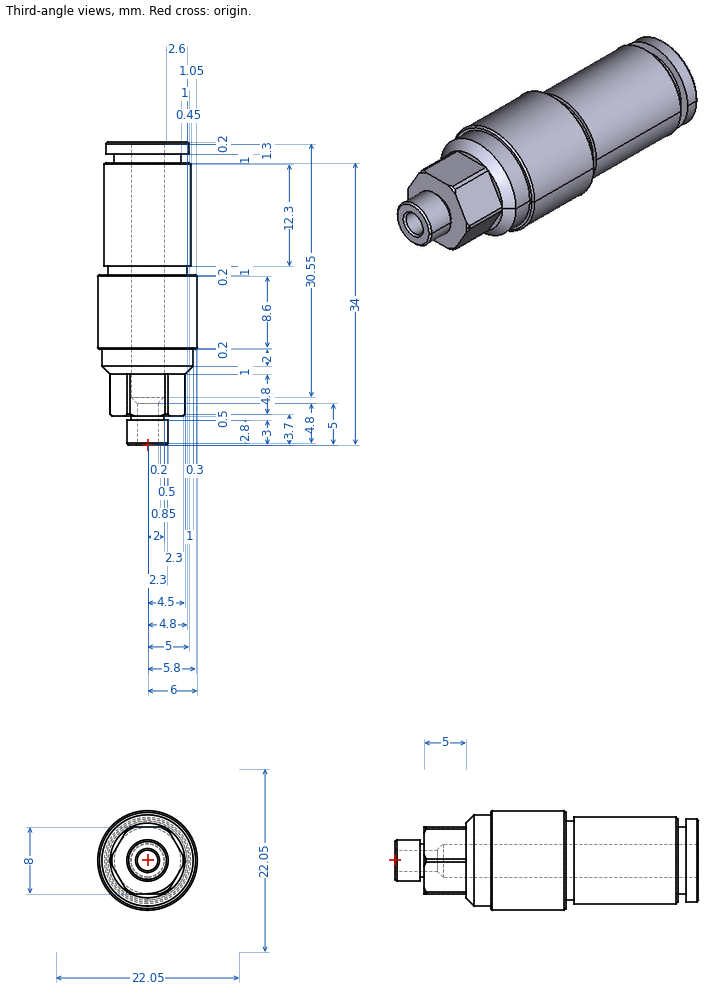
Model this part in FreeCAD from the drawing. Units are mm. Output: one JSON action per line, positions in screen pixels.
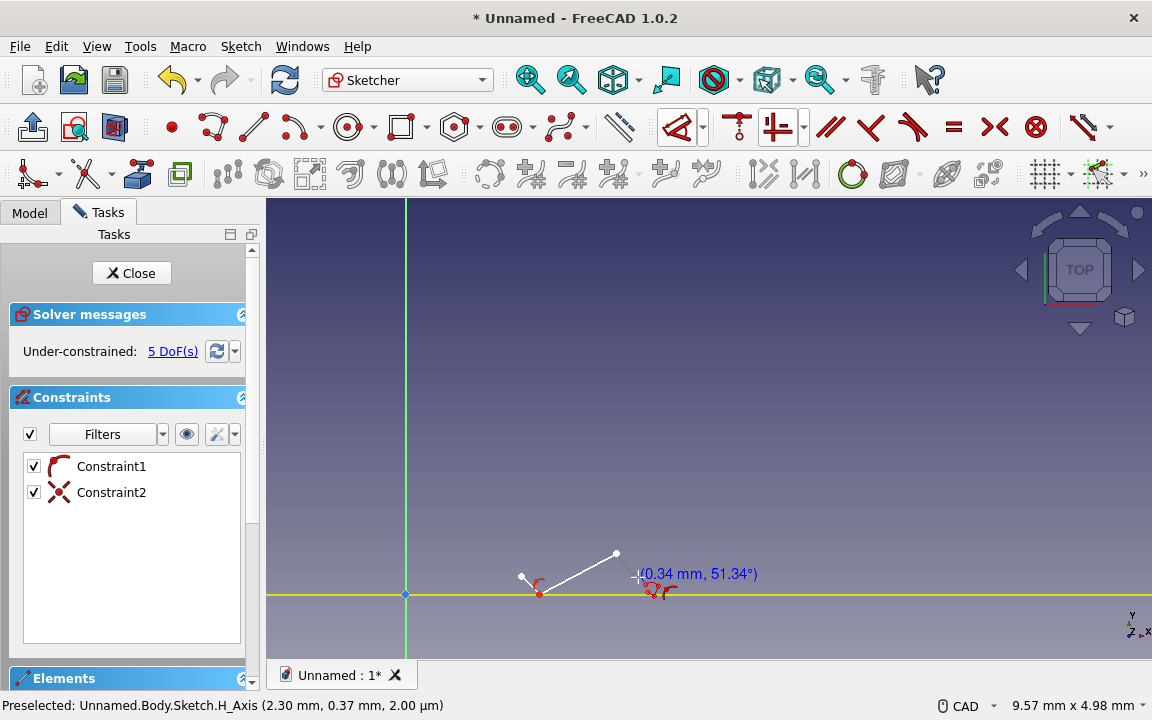
{"action": "left_click", "coordinate": [637, 576]}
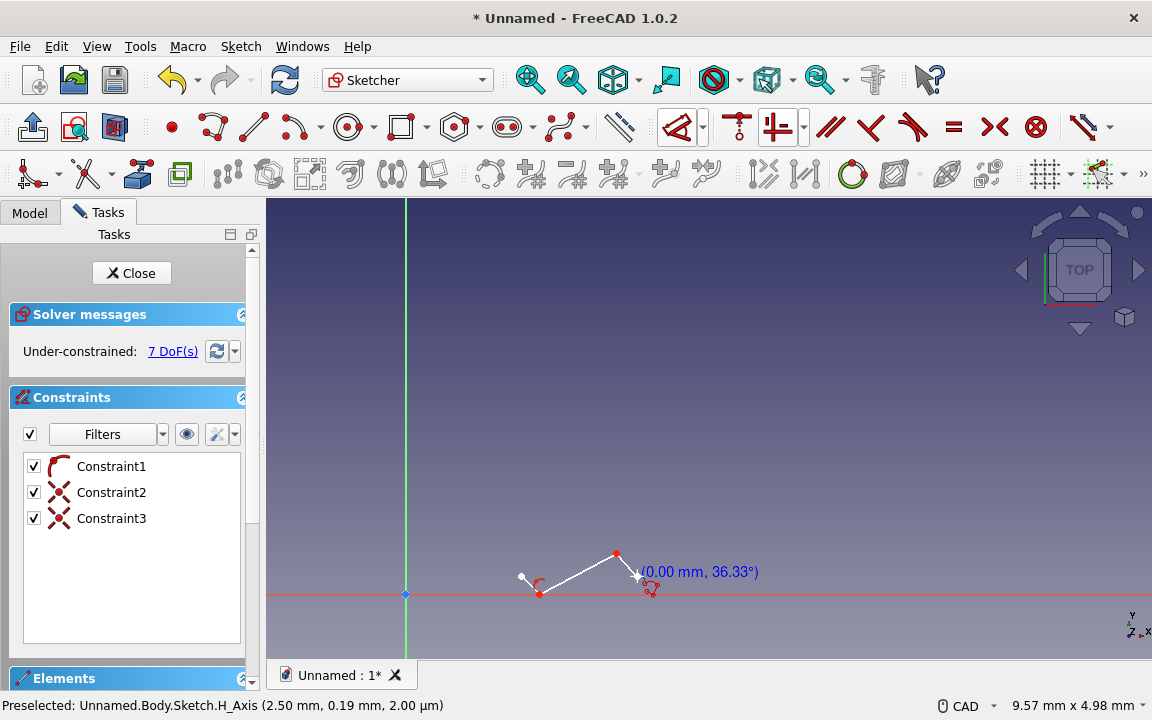
{"action": "scroll", "coordinate": [636, 581], "scroll_direction": "down", "scroll_amount": 12}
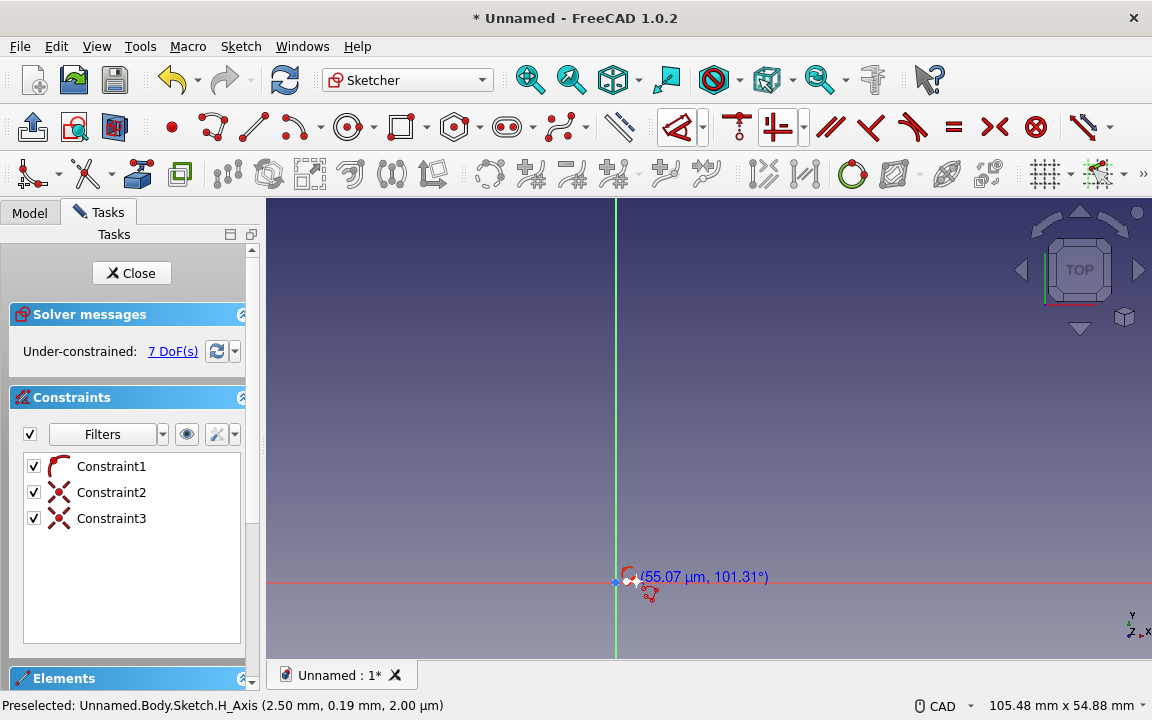
{"action": "left_click", "coordinate": [636, 558]}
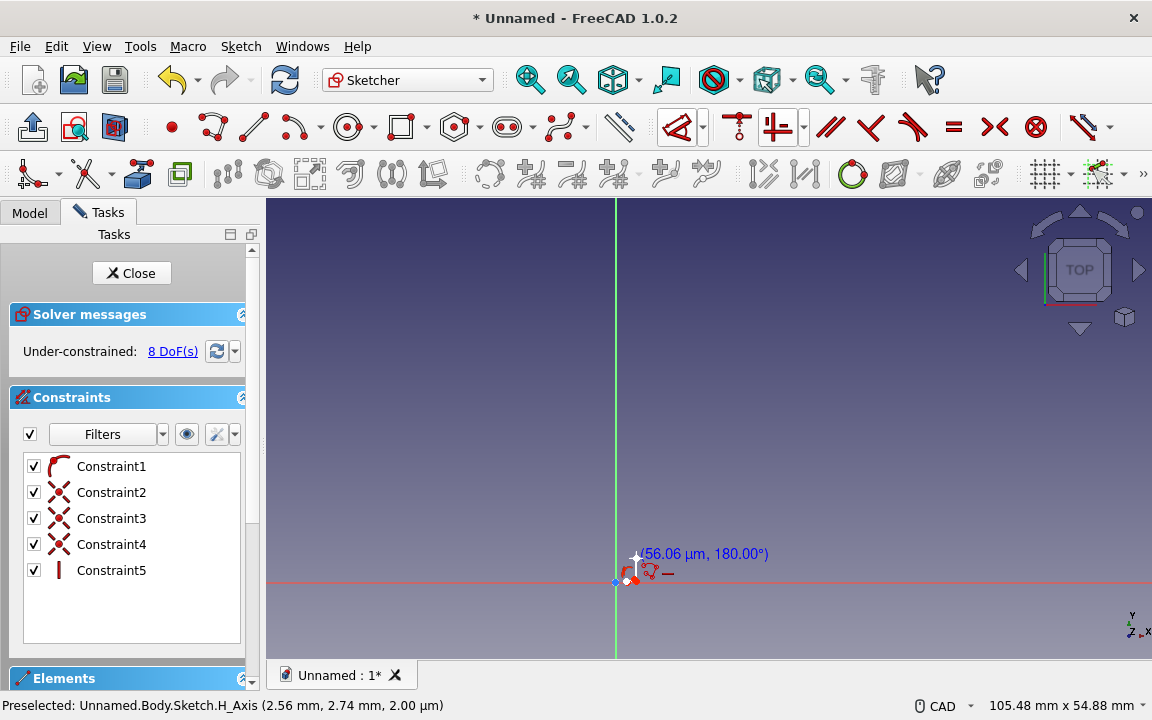
{"action": "scroll", "coordinate": [632, 558], "scroll_direction": "up", "scroll_amount": 7}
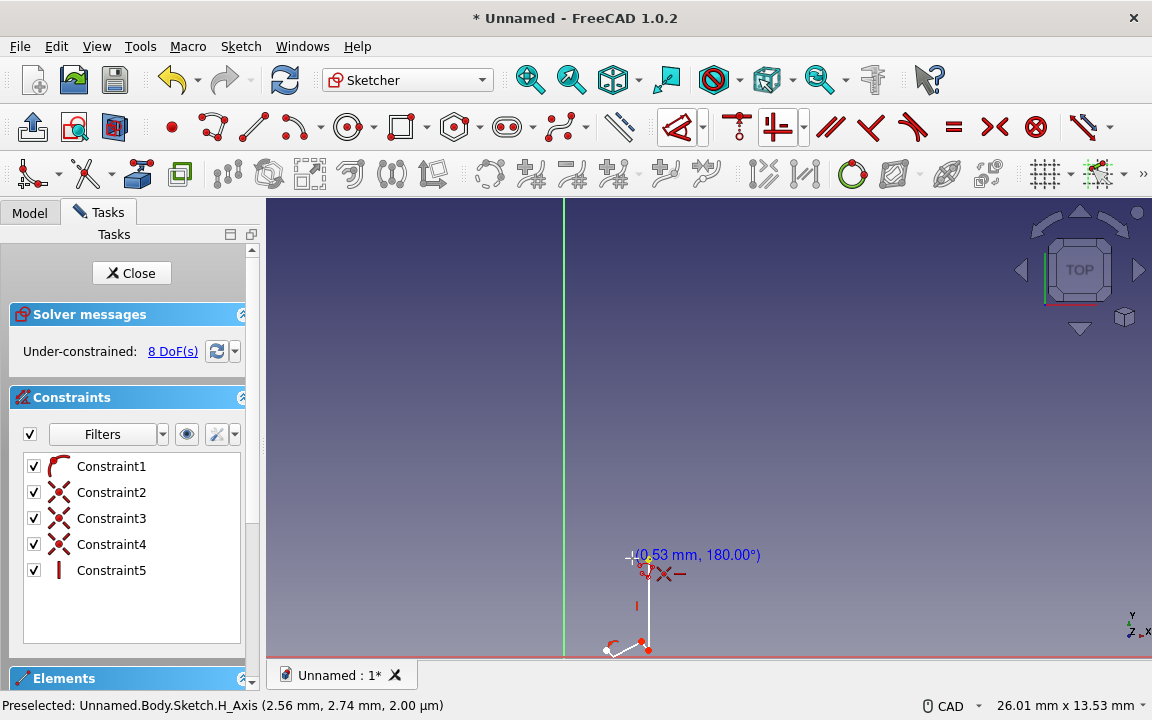
{"action": "left_click", "coordinate": [632, 556]}
{"action": "left_click", "coordinate": [632, 538]}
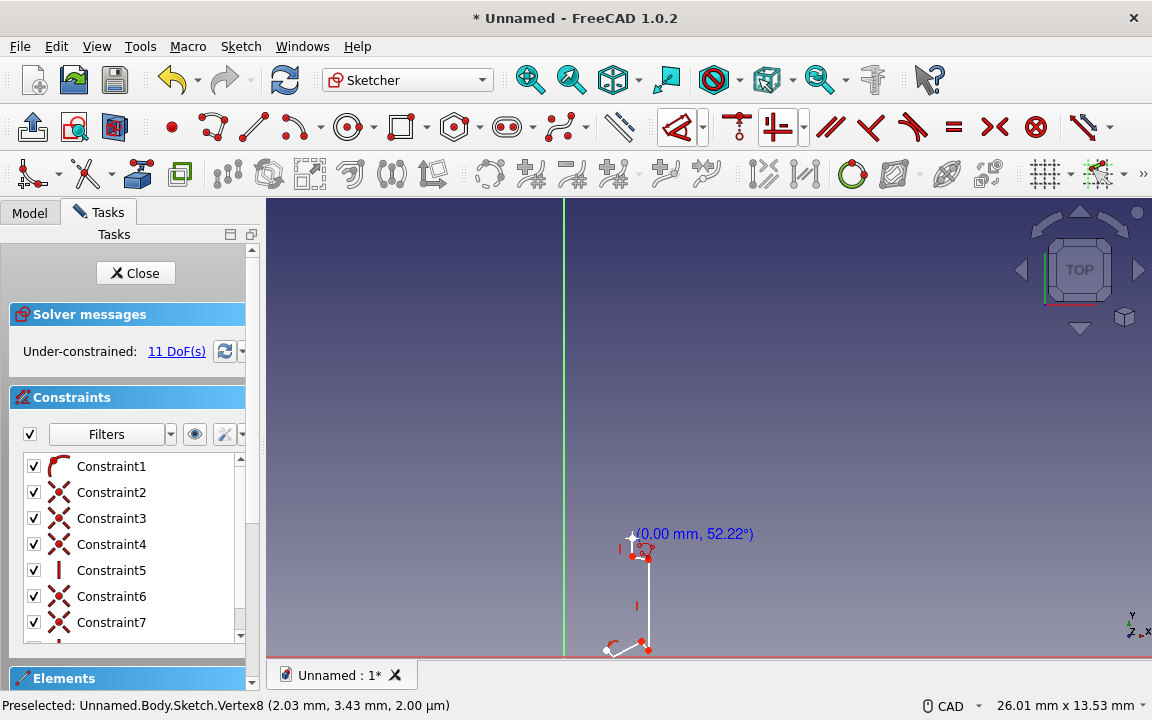
{"action": "scroll", "coordinate": [632, 557], "scroll_direction": "down", "scroll_amount": 7}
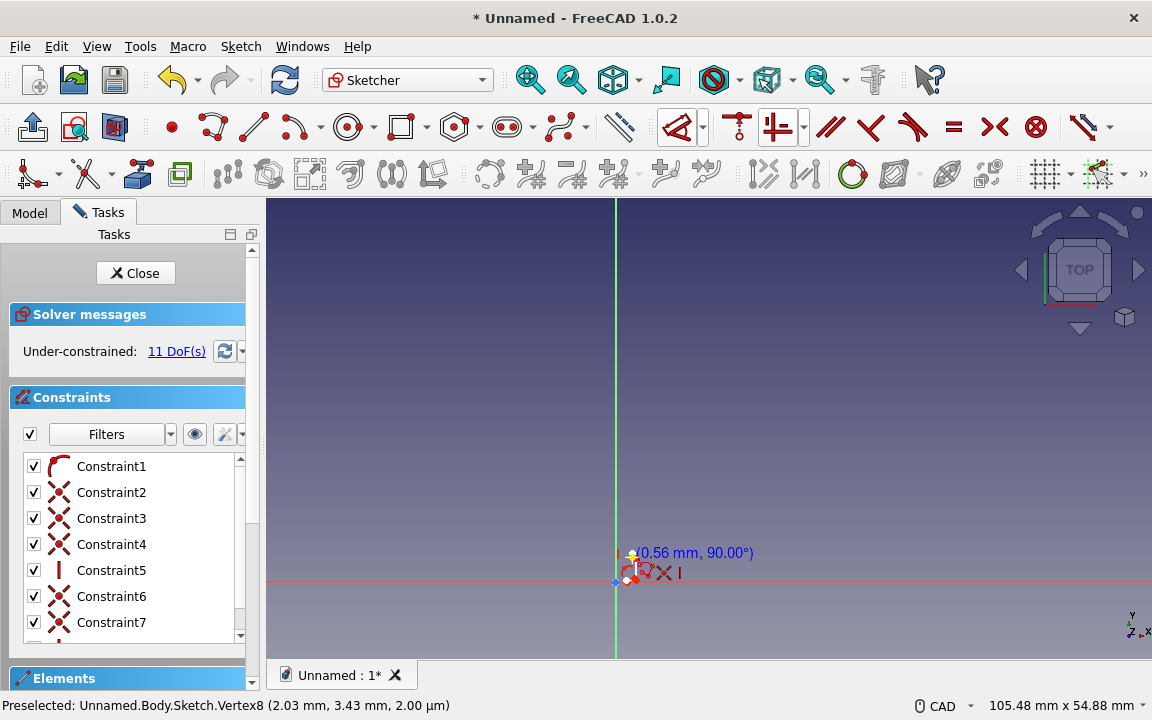
{"action": "left_click", "coordinate": [652, 553]}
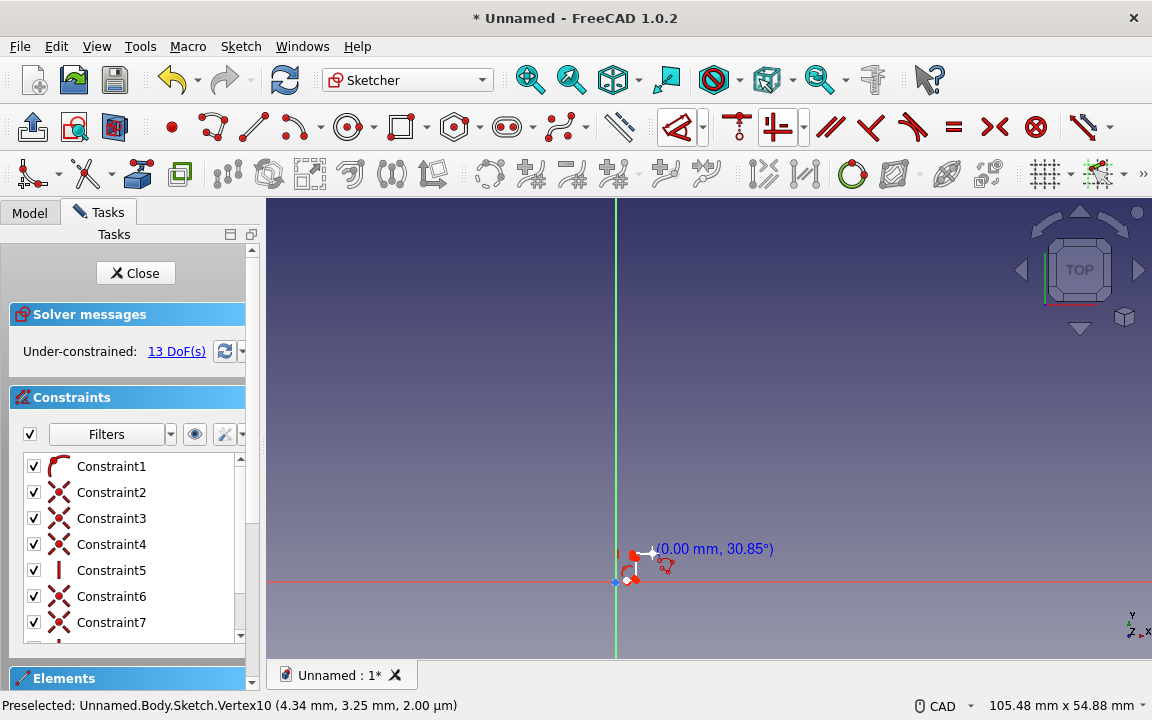
{"action": "scroll", "coordinate": [653, 551], "scroll_direction": "up", "scroll_amount": 10}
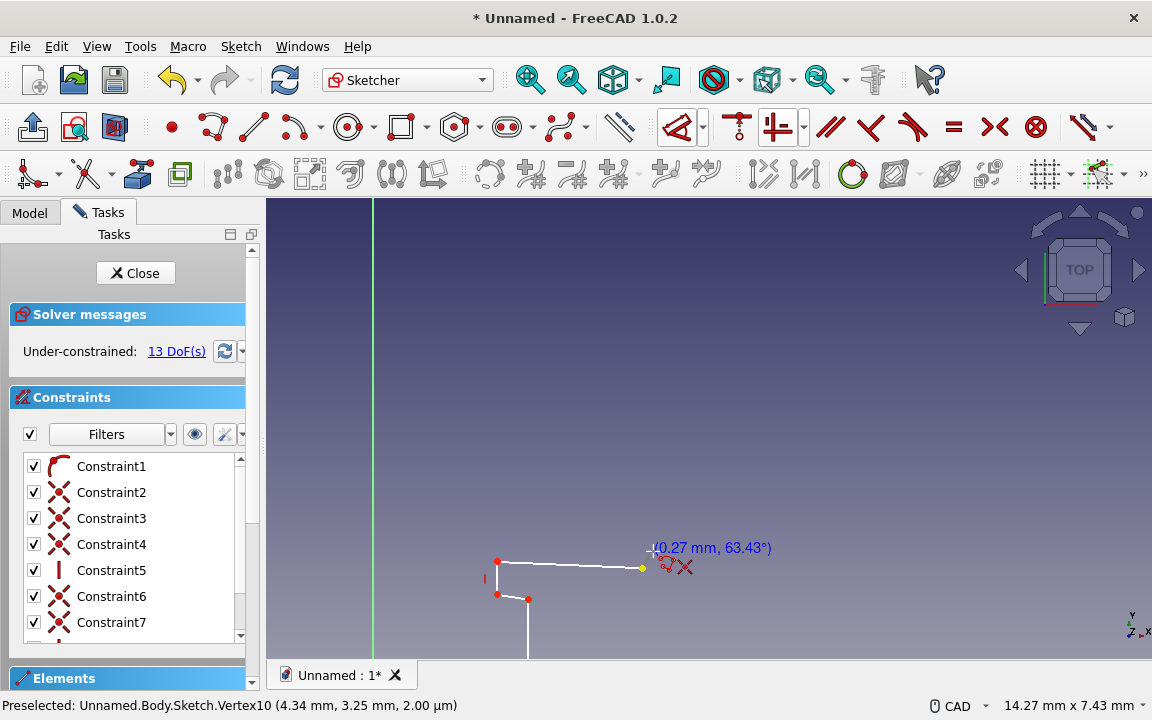
{"action": "left_click", "coordinate": [652, 547]}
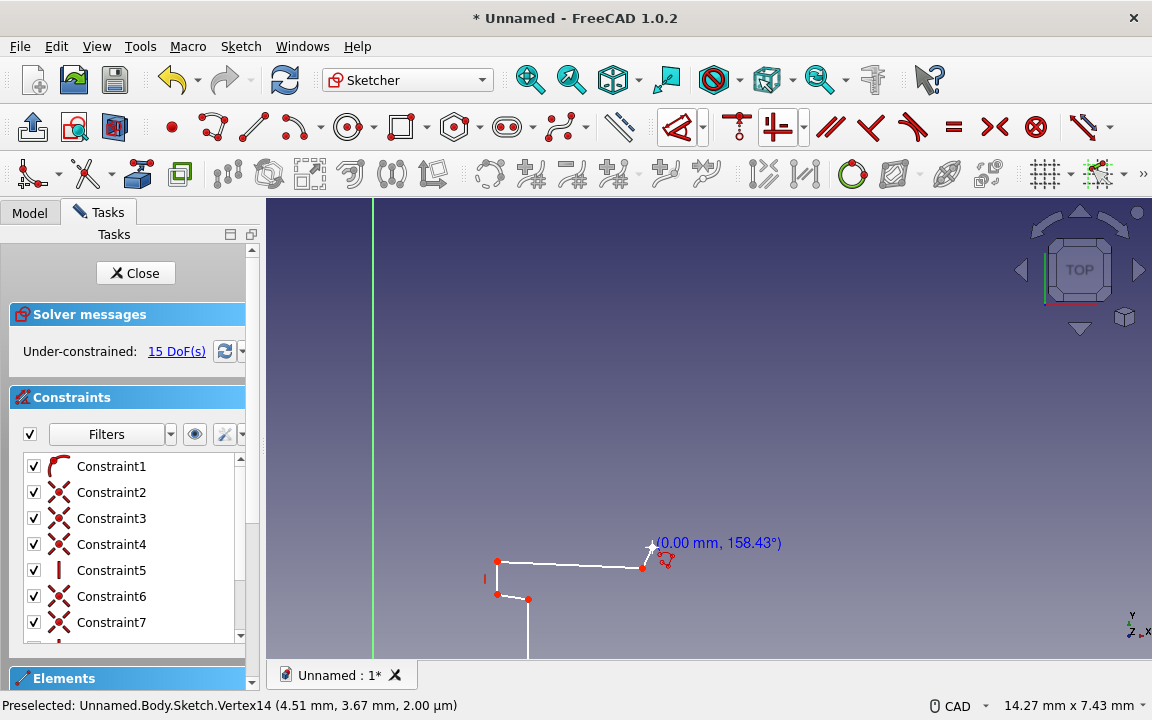
{"action": "scroll", "coordinate": [653, 551], "scroll_direction": "down", "scroll_amount": 10}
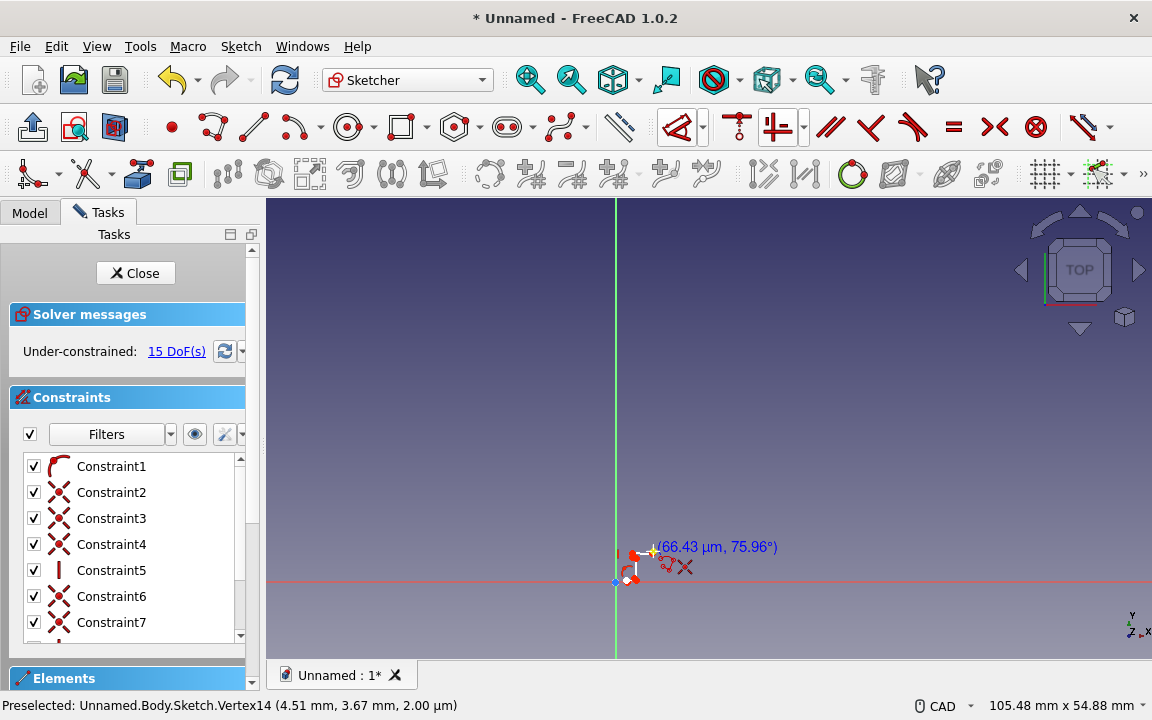
{"action": "left_click", "coordinate": [653, 511]}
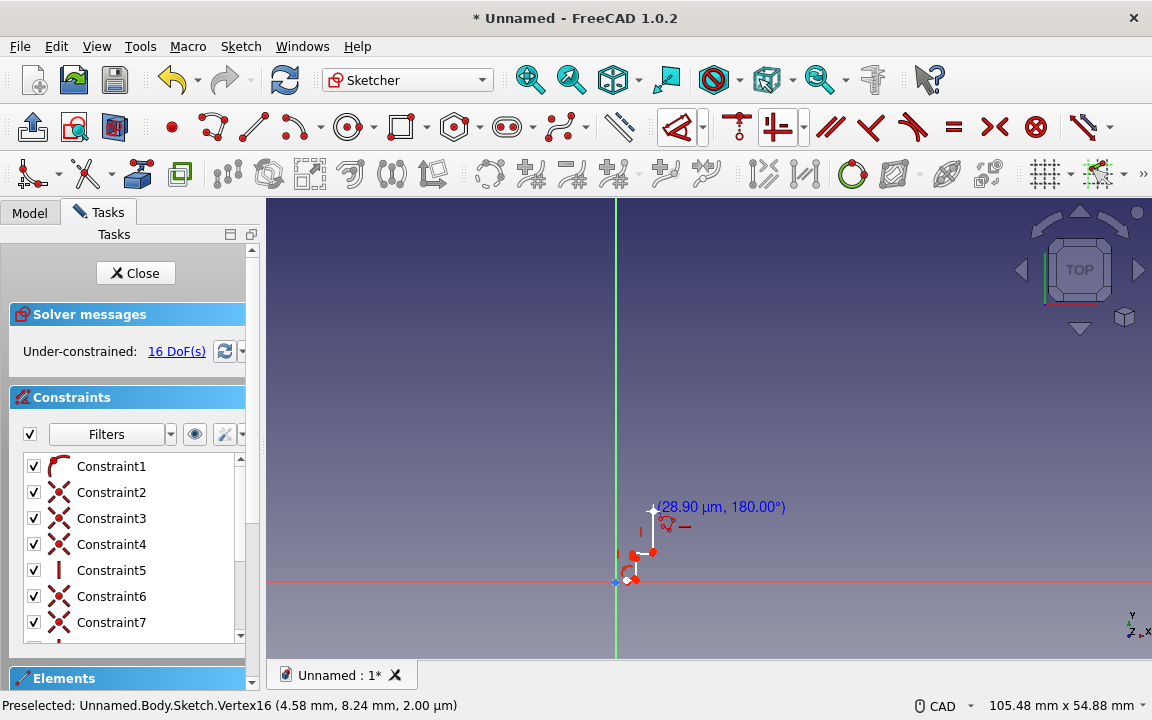
{"action": "scroll", "coordinate": [662, 502], "scroll_direction": "up", "scroll_amount": 2}